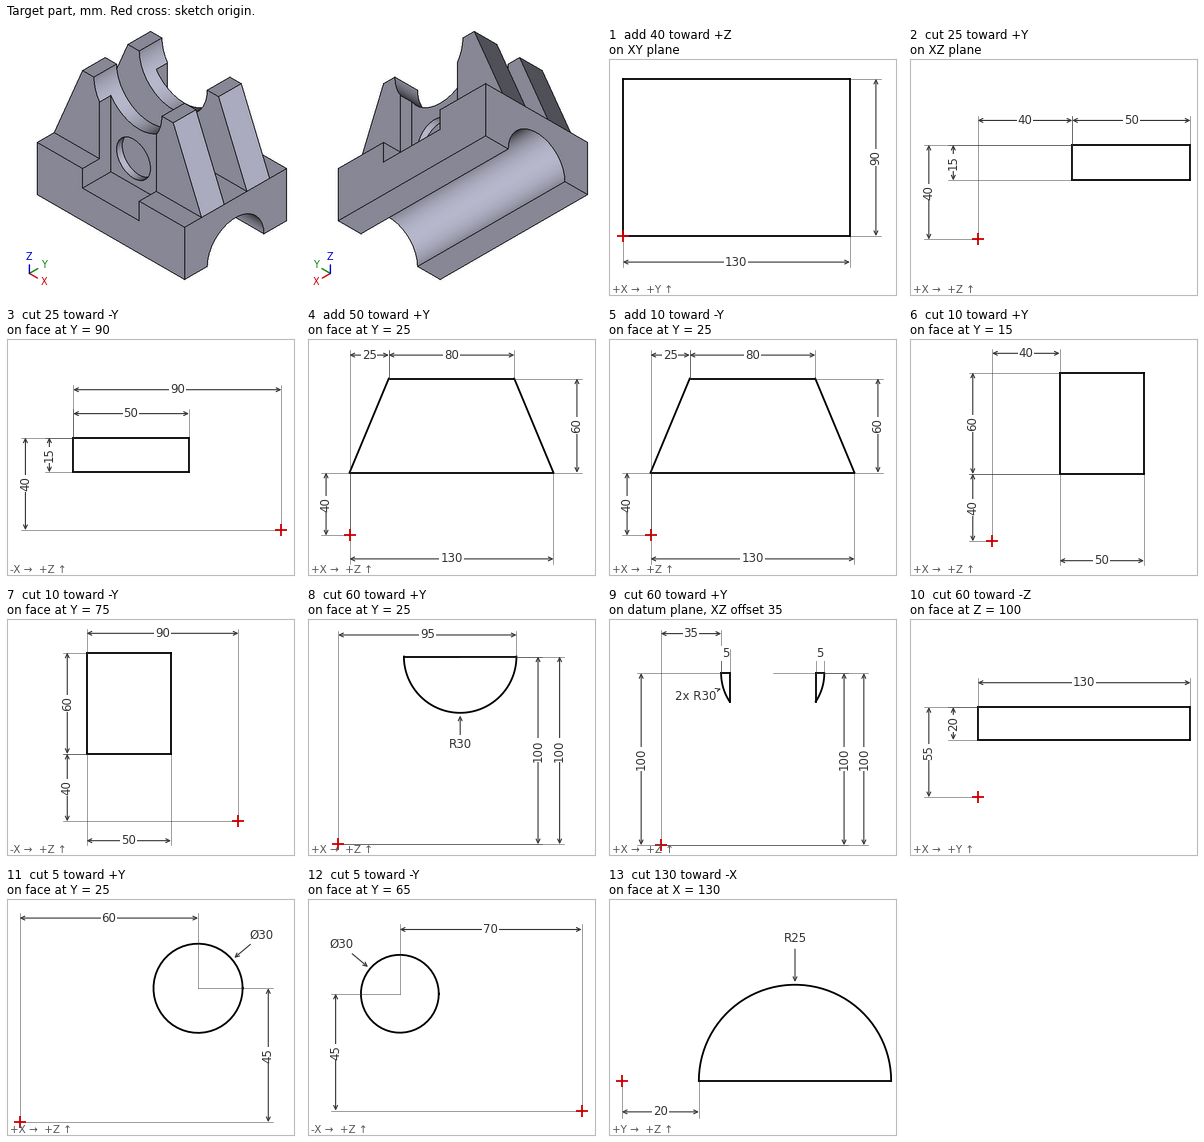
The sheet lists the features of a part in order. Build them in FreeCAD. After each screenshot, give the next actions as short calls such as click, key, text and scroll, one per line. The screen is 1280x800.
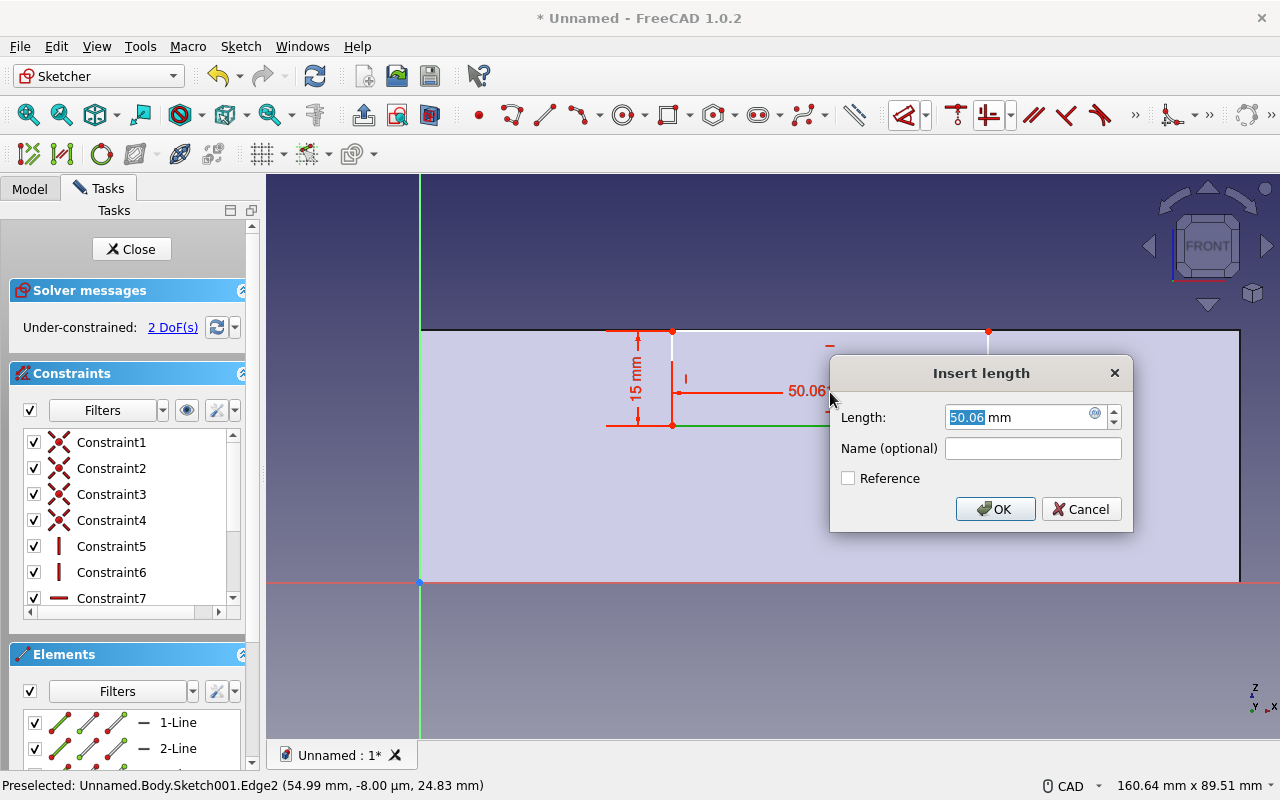
text(50)
key(Return)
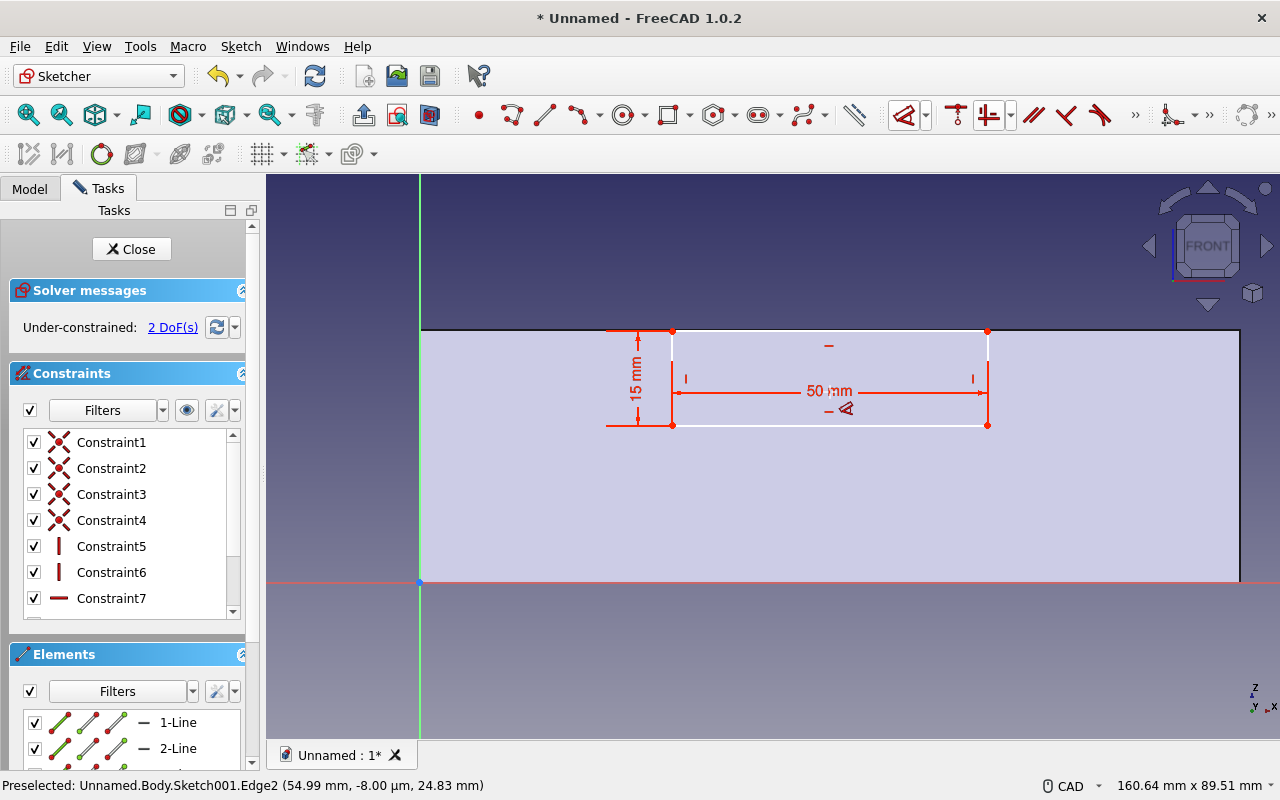
click(672, 331)
click(546, 617)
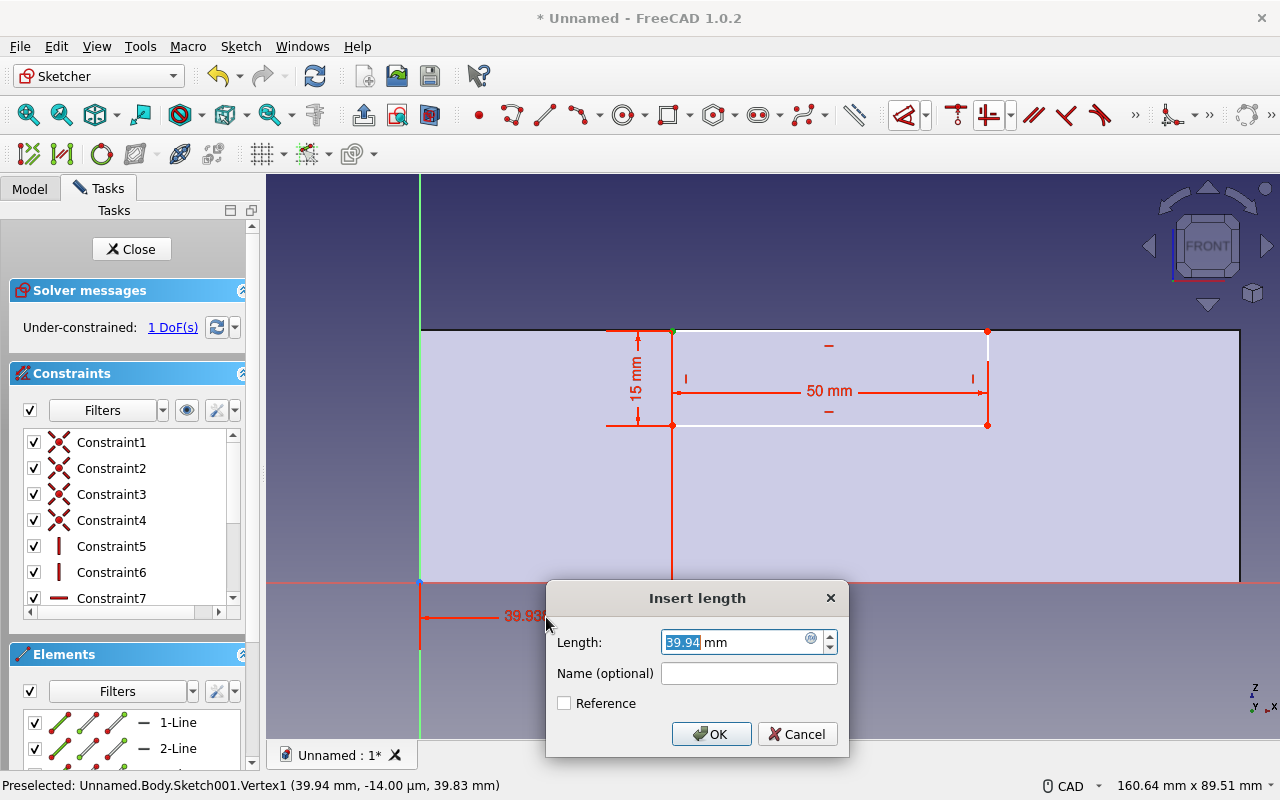
text(40)
key(Return)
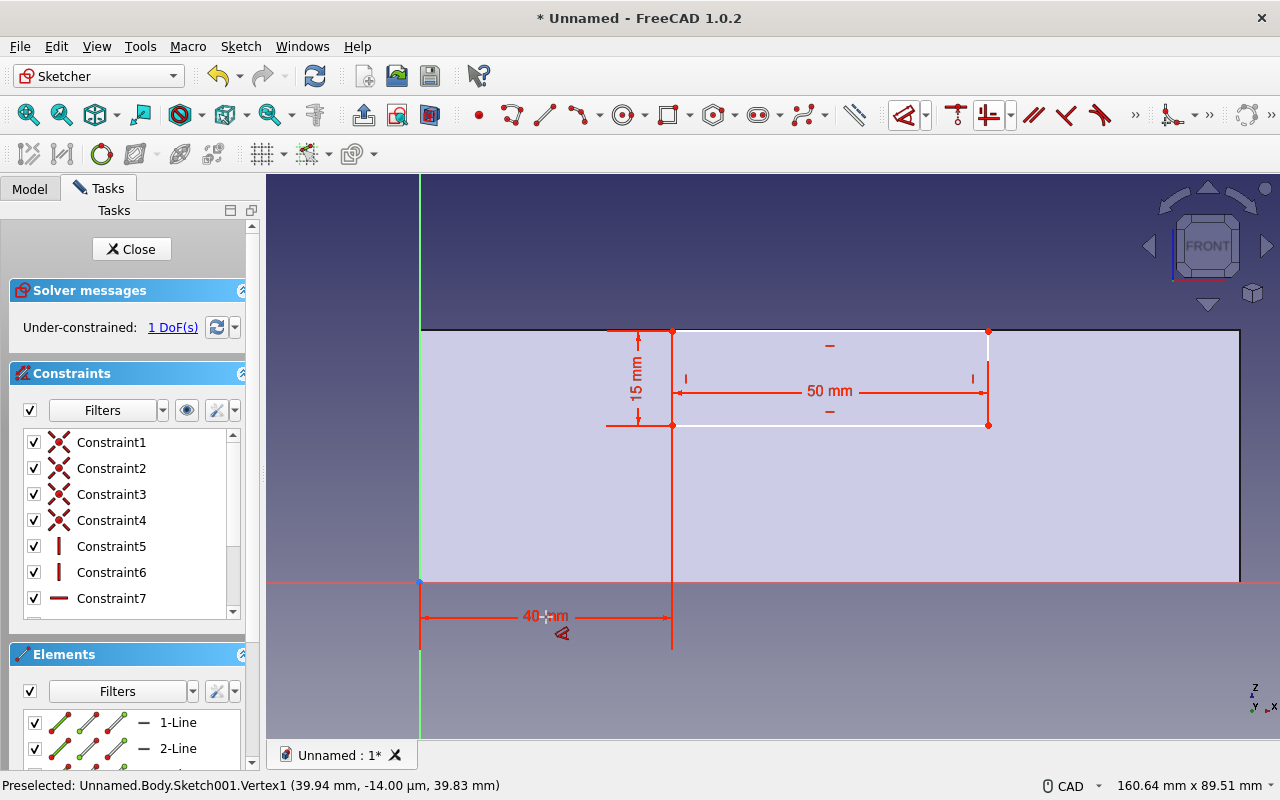
click(672, 331)
click(386, 457)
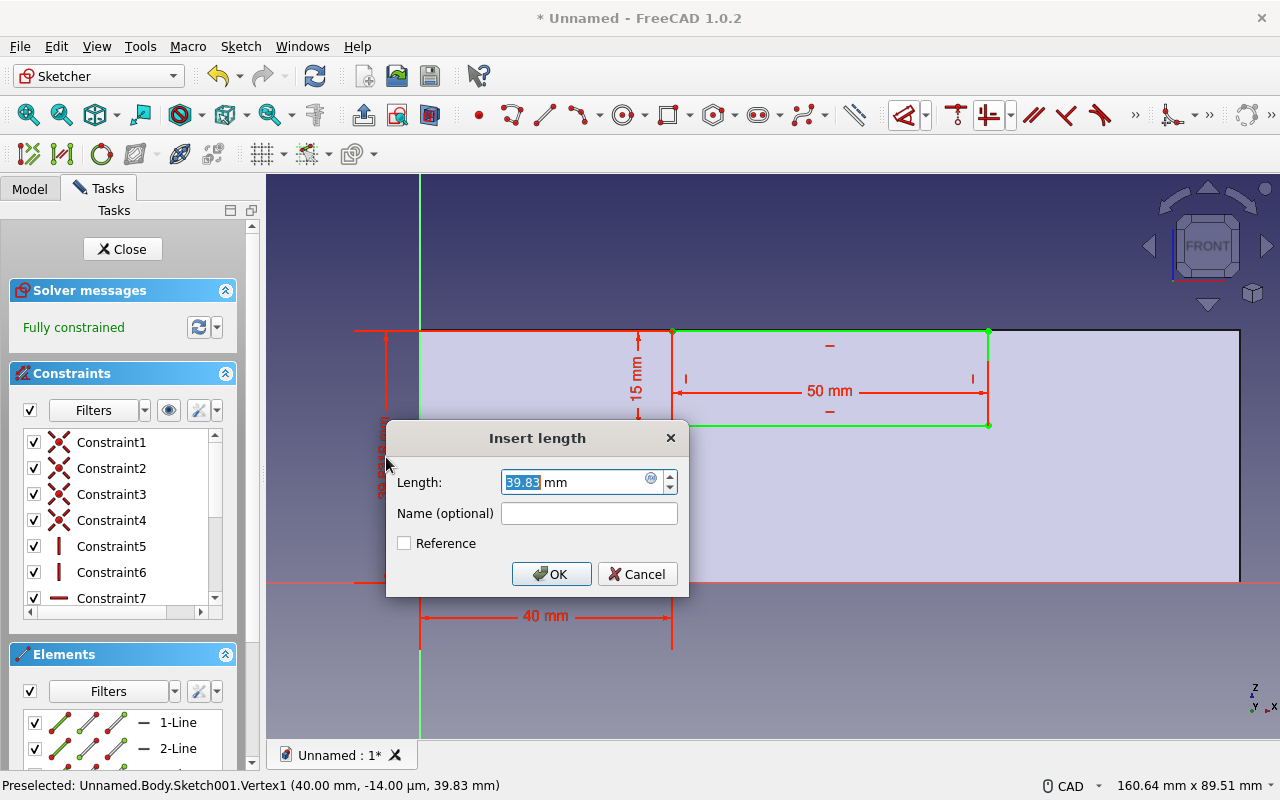
text(40)
key(Return)
key(Escape)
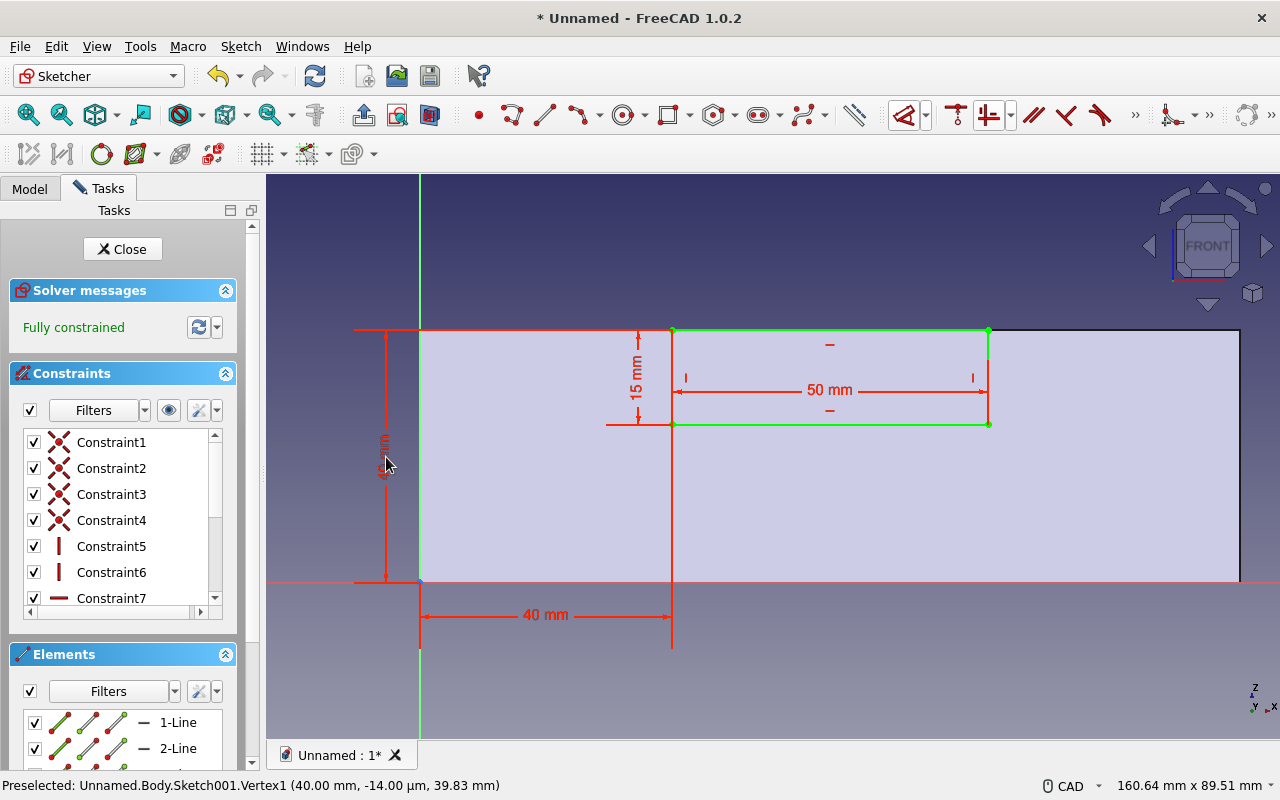
click(123, 249)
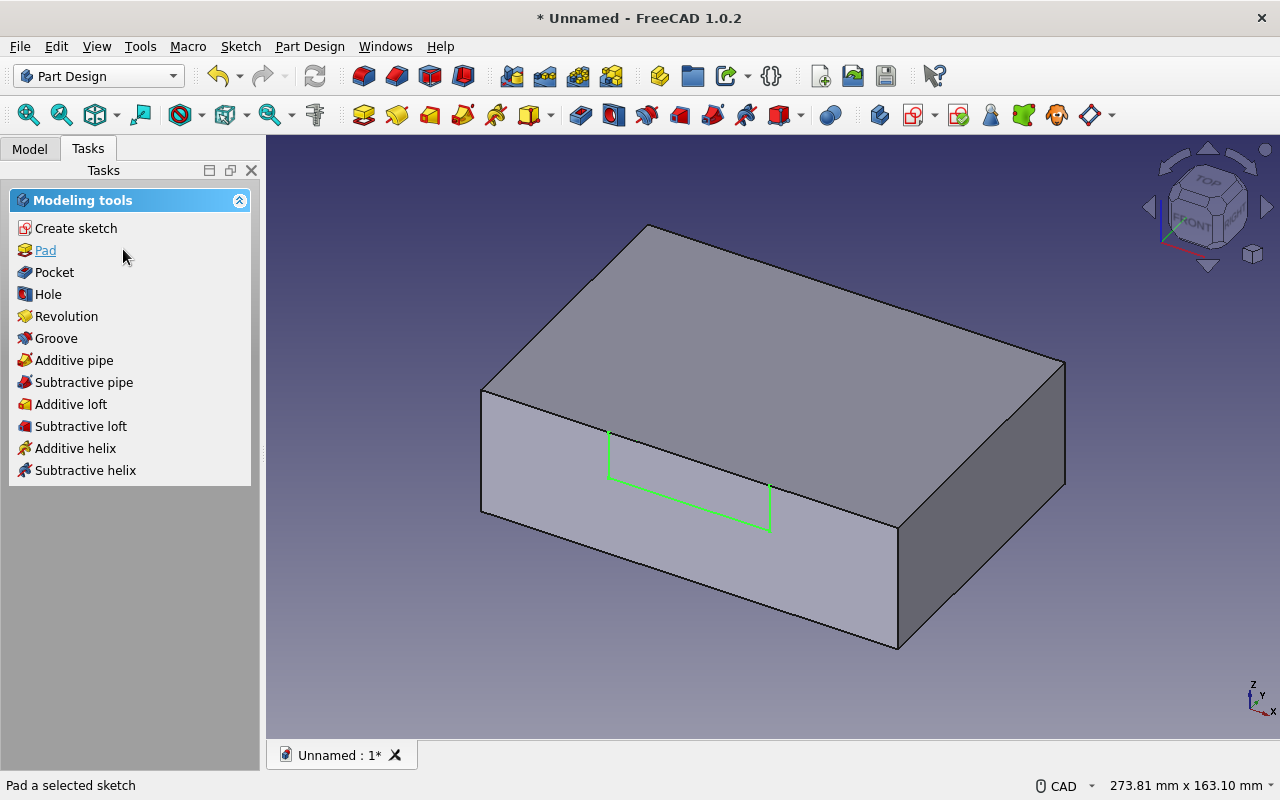
click(581, 116)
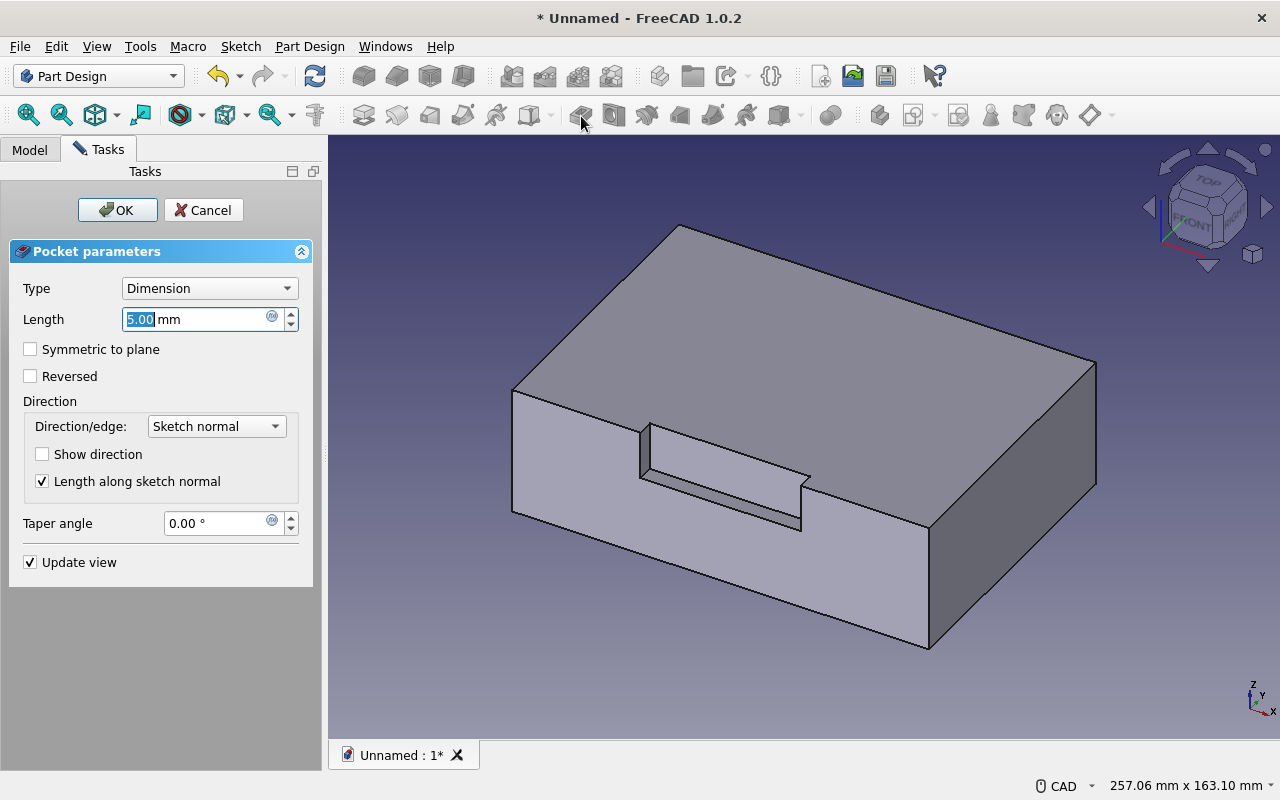
text(25)
key(Tab)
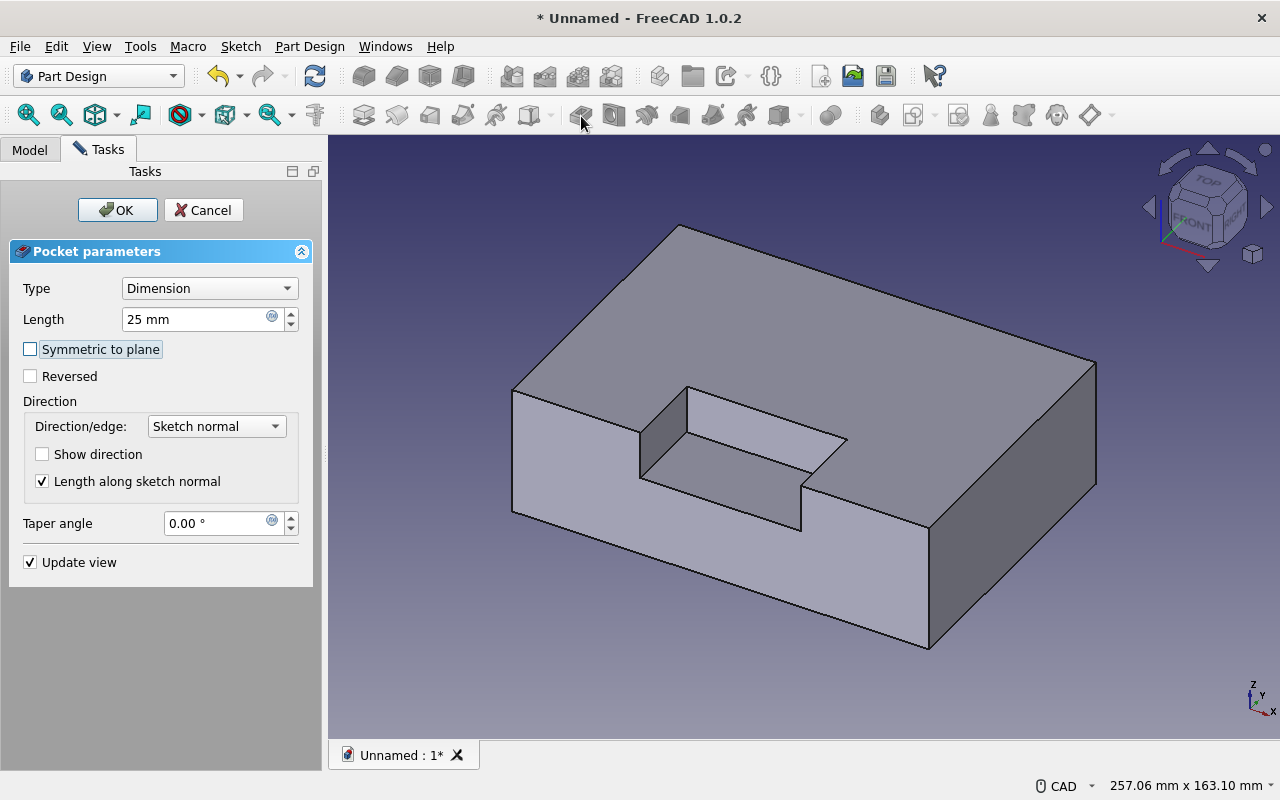
click(118, 210)